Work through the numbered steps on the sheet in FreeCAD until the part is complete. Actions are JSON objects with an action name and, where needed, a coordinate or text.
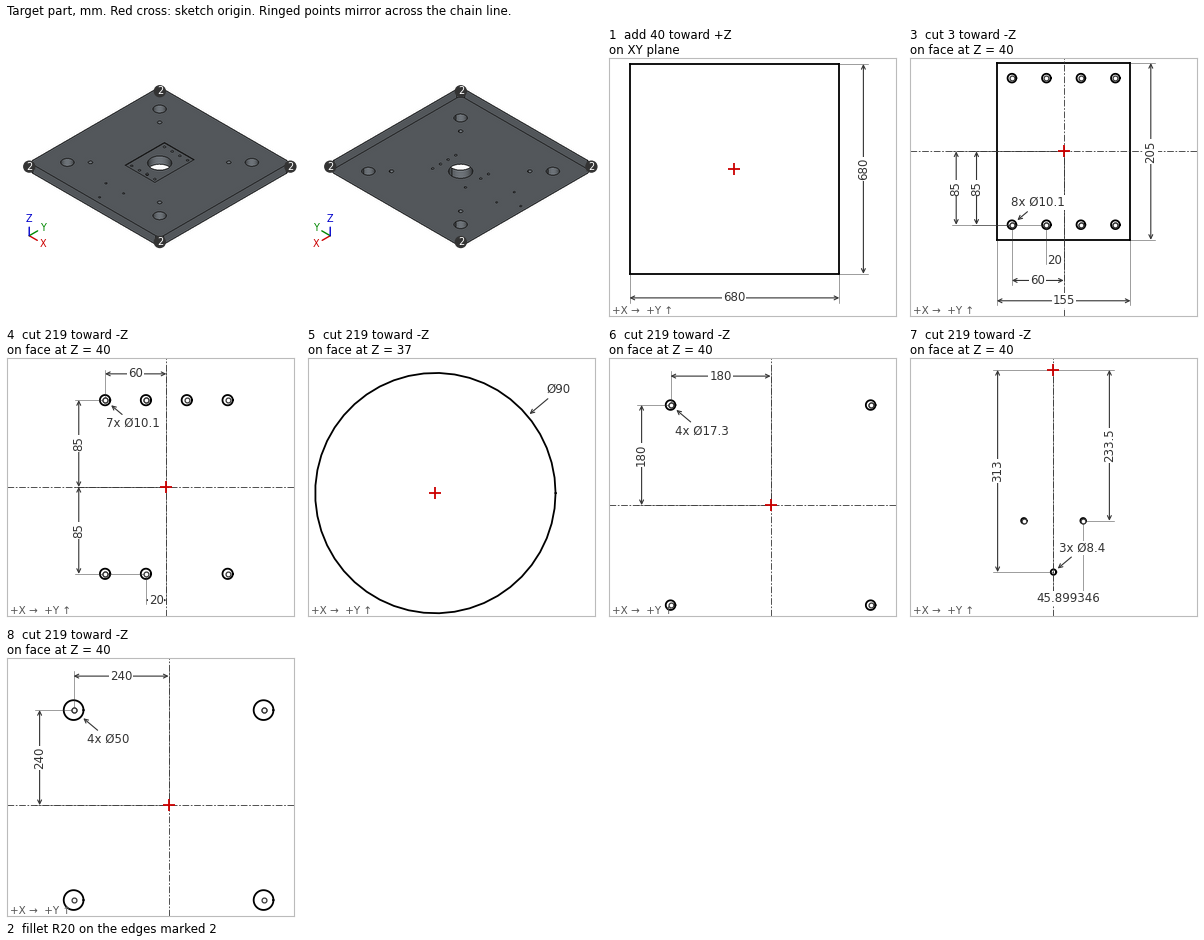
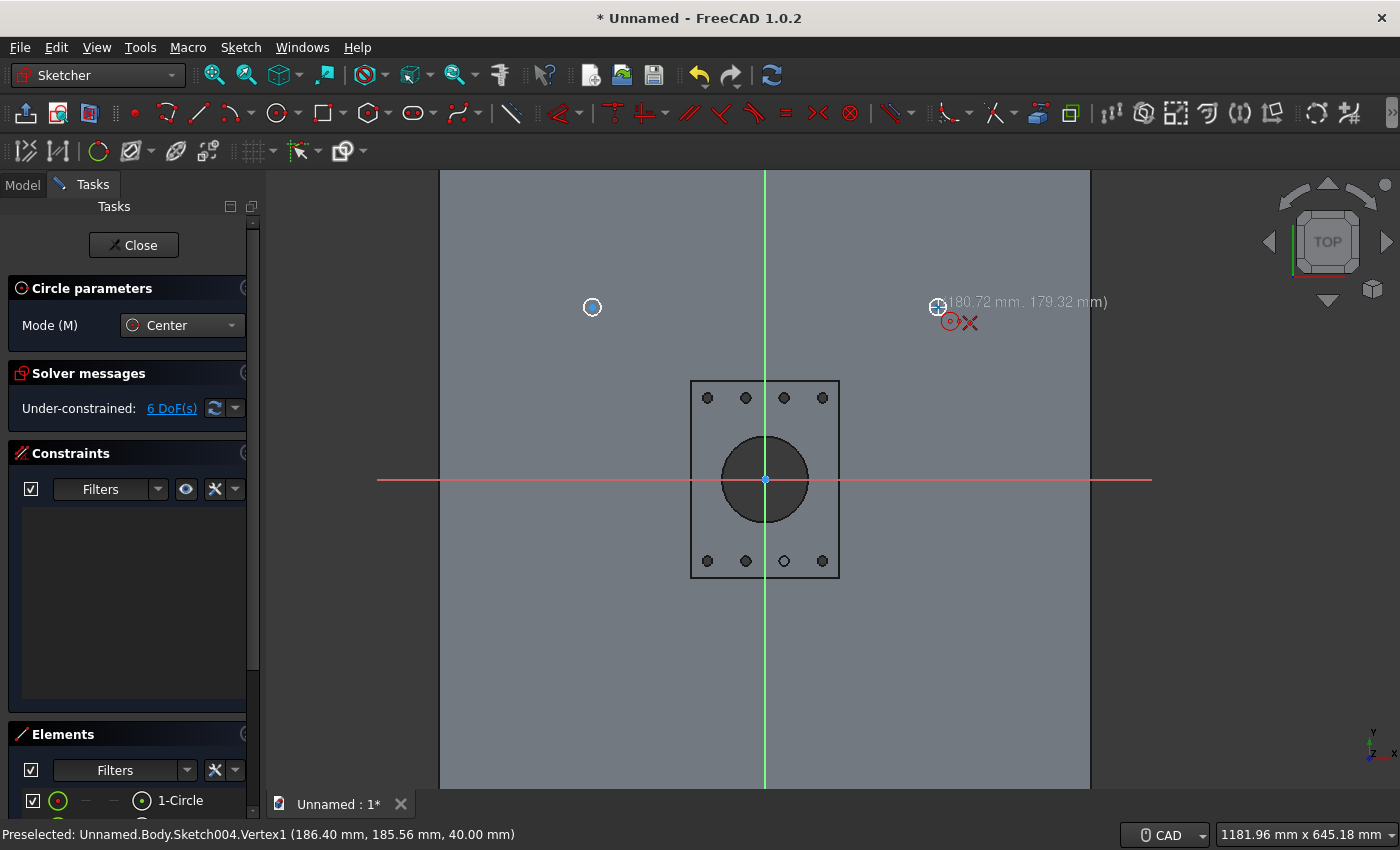
{"action": "scroll", "coordinate": [938, 652], "scroll_direction": "up", "scroll_amount": 6}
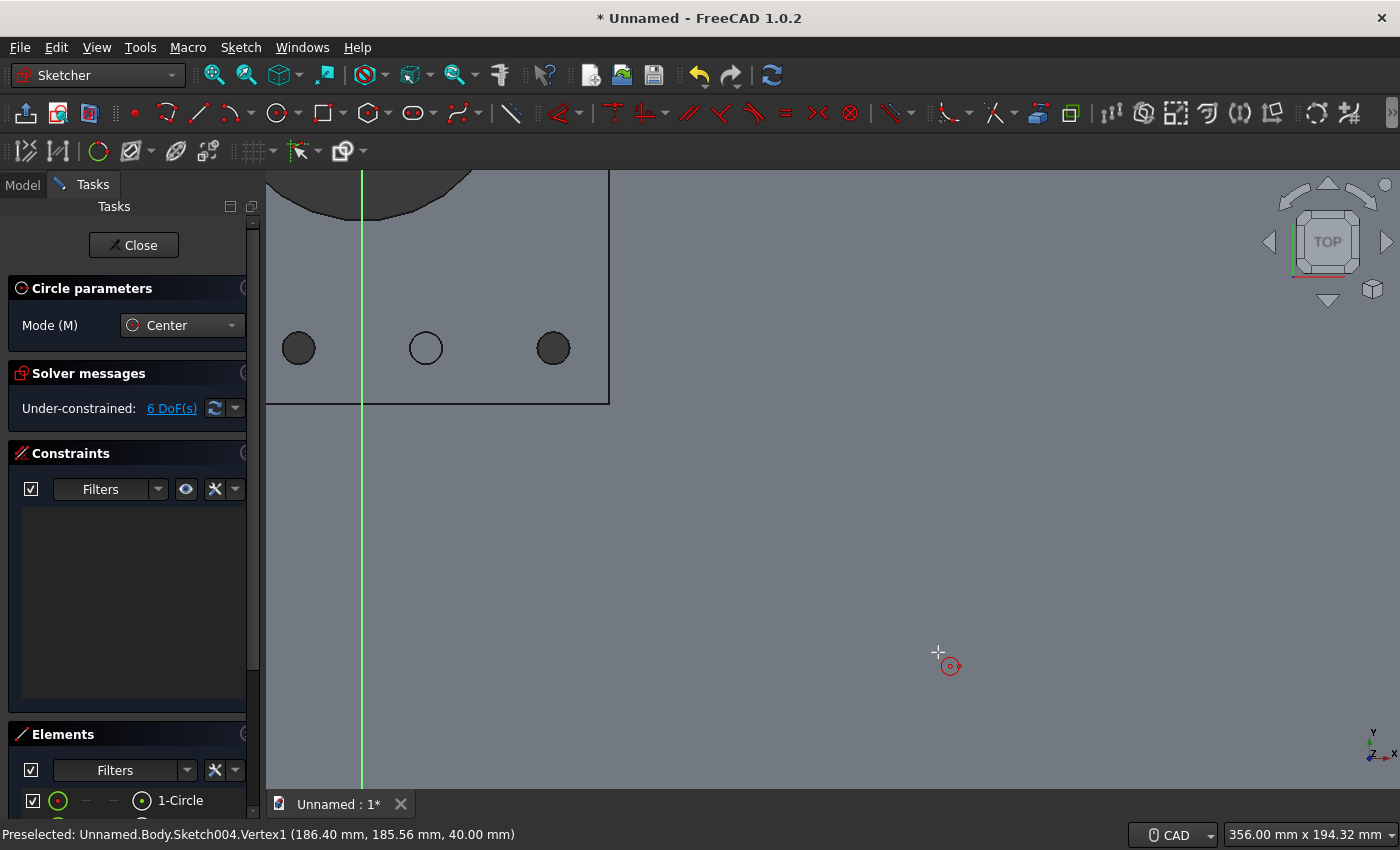
{"action": "left_click", "coordinate": [936, 651]}
{"action": "left_click", "coordinate": [955, 631]}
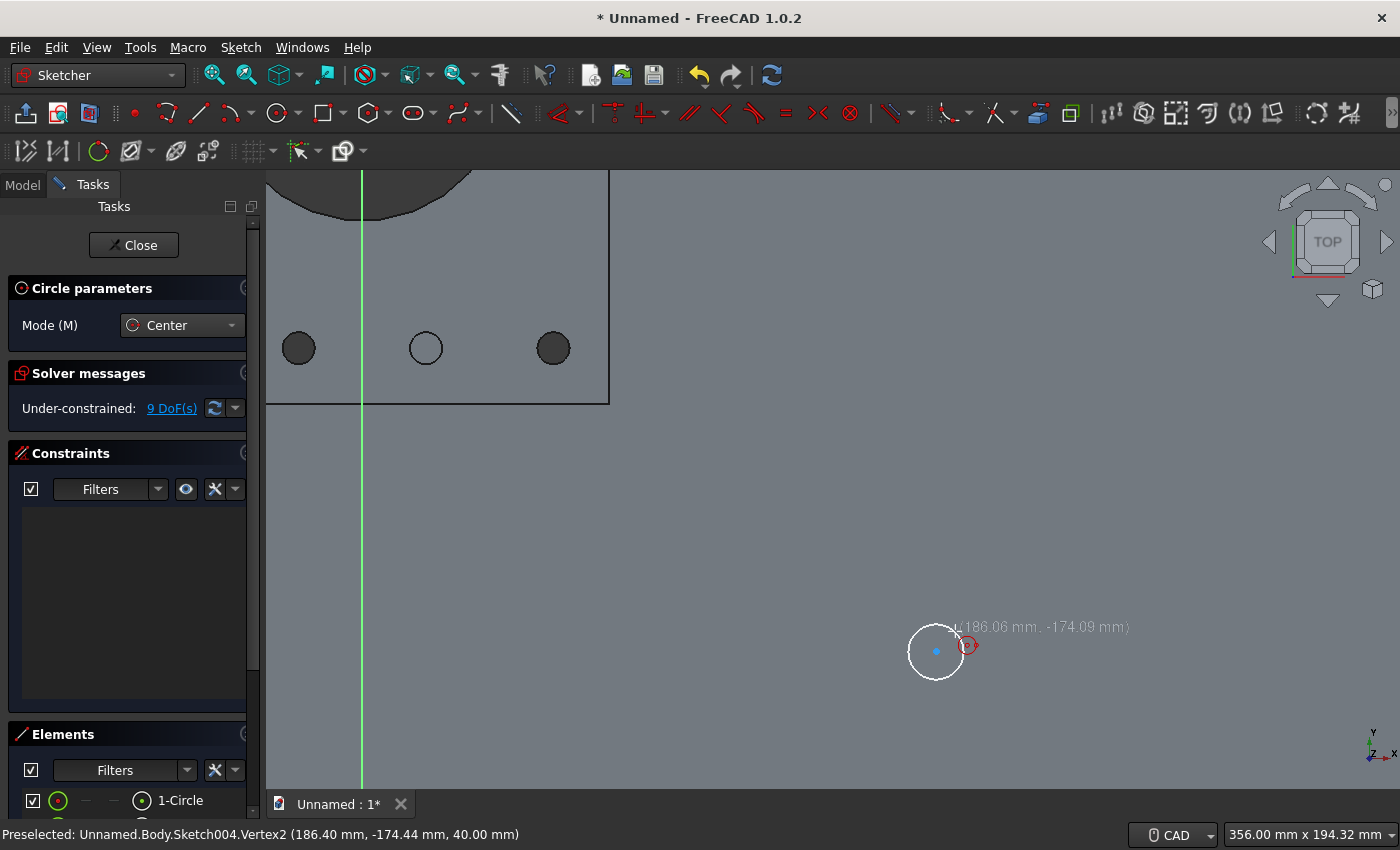
{"action": "scroll", "coordinate": [938, 653], "scroll_direction": "down", "scroll_amount": 6}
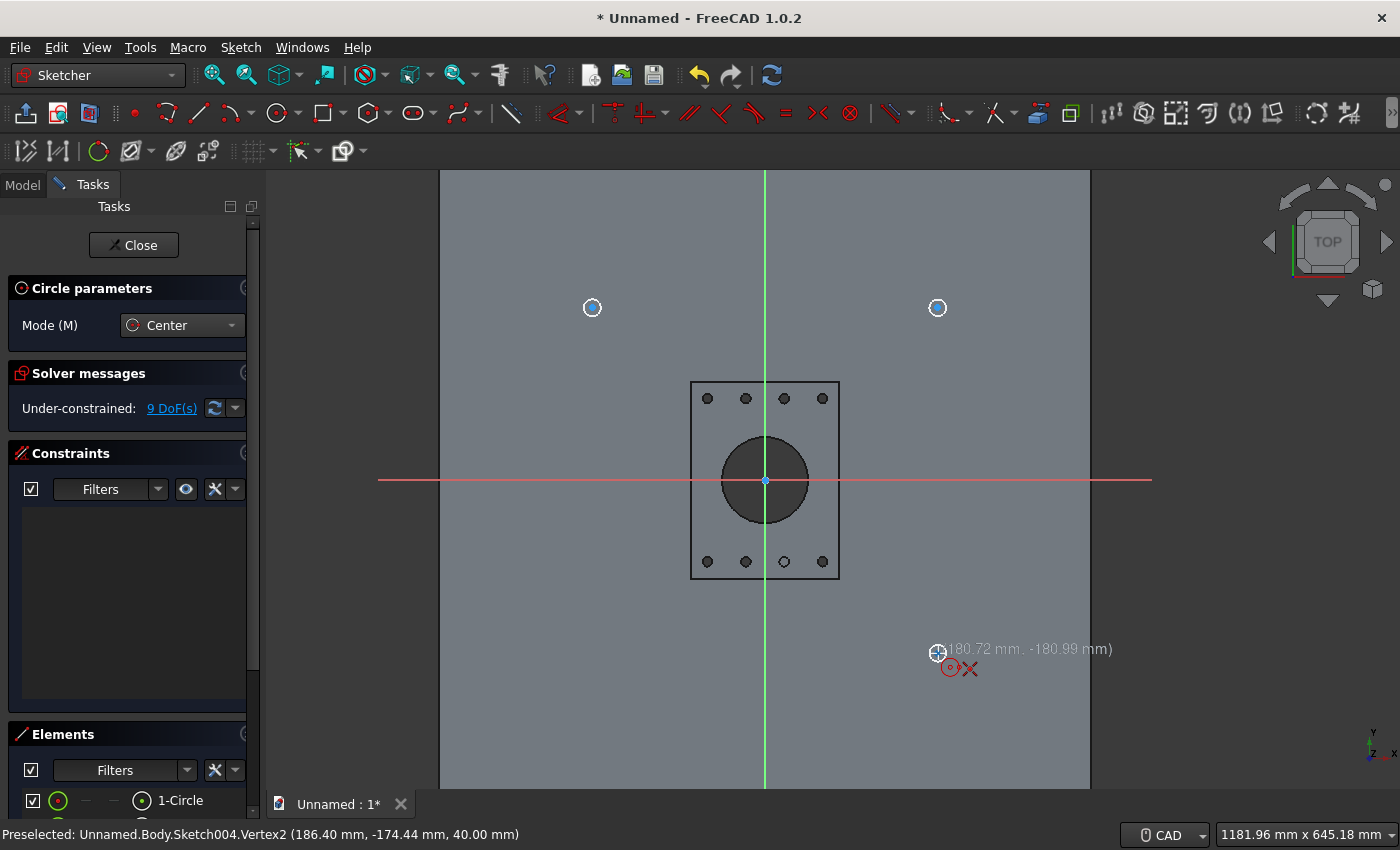
{"action": "scroll", "coordinate": [592, 653], "scroll_direction": "up", "scroll_amount": 6}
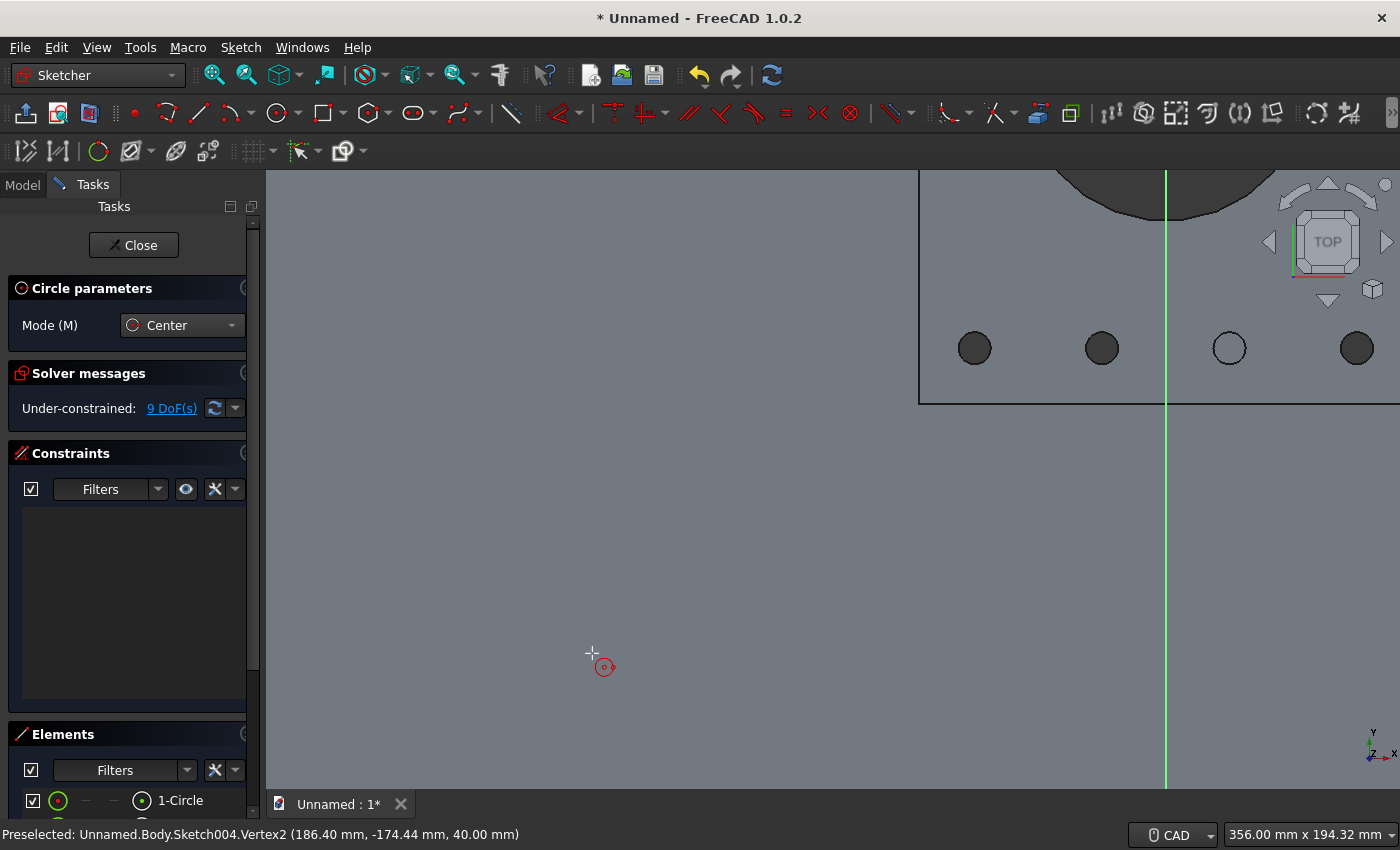
{"action": "left_click", "coordinate": [592, 651]}
{"action": "left_click", "coordinate": [612, 631]}
{"action": "key", "text": "Escape"}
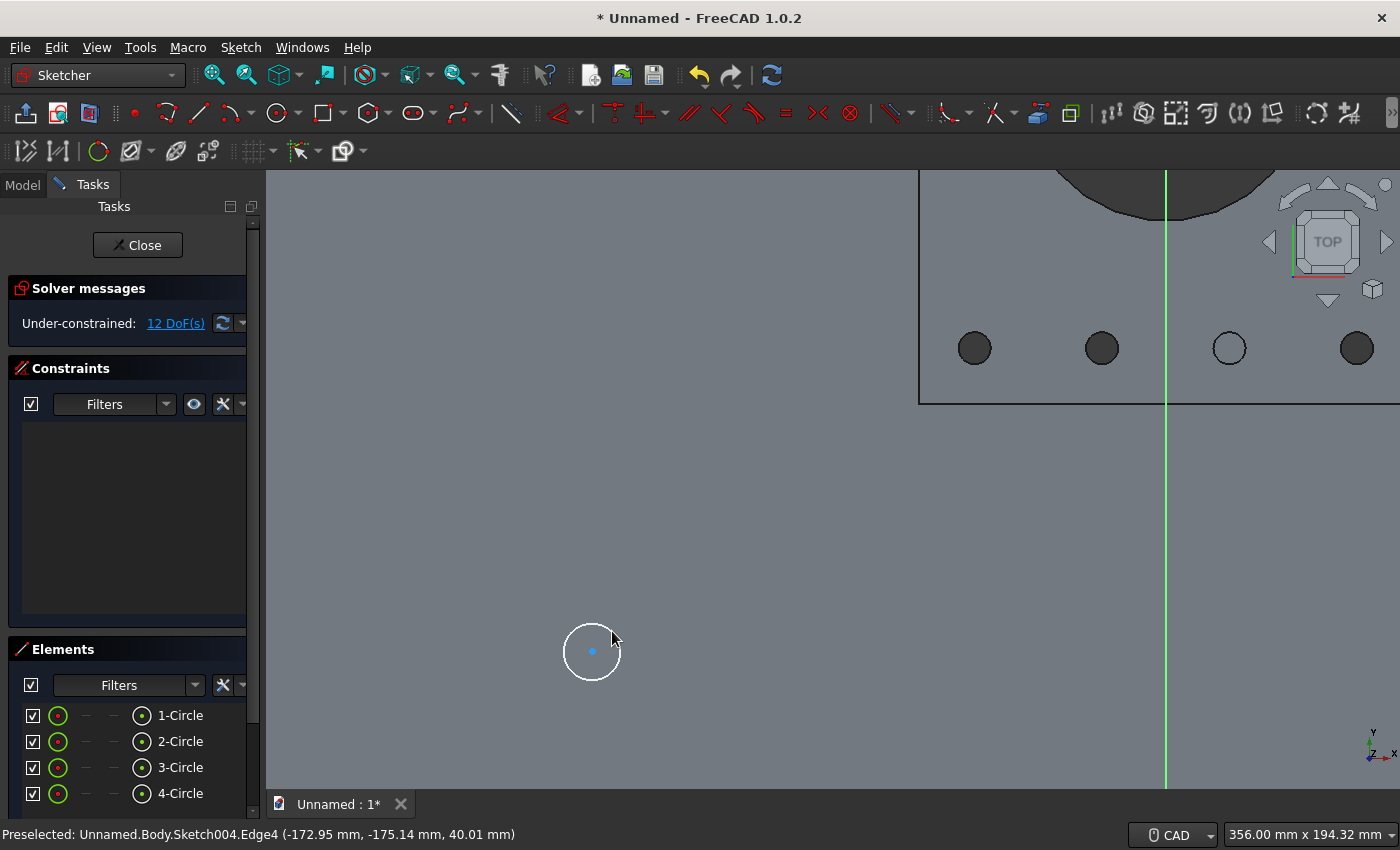
{"action": "scroll", "coordinate": [592, 653], "scroll_direction": "down", "scroll_amount": 6}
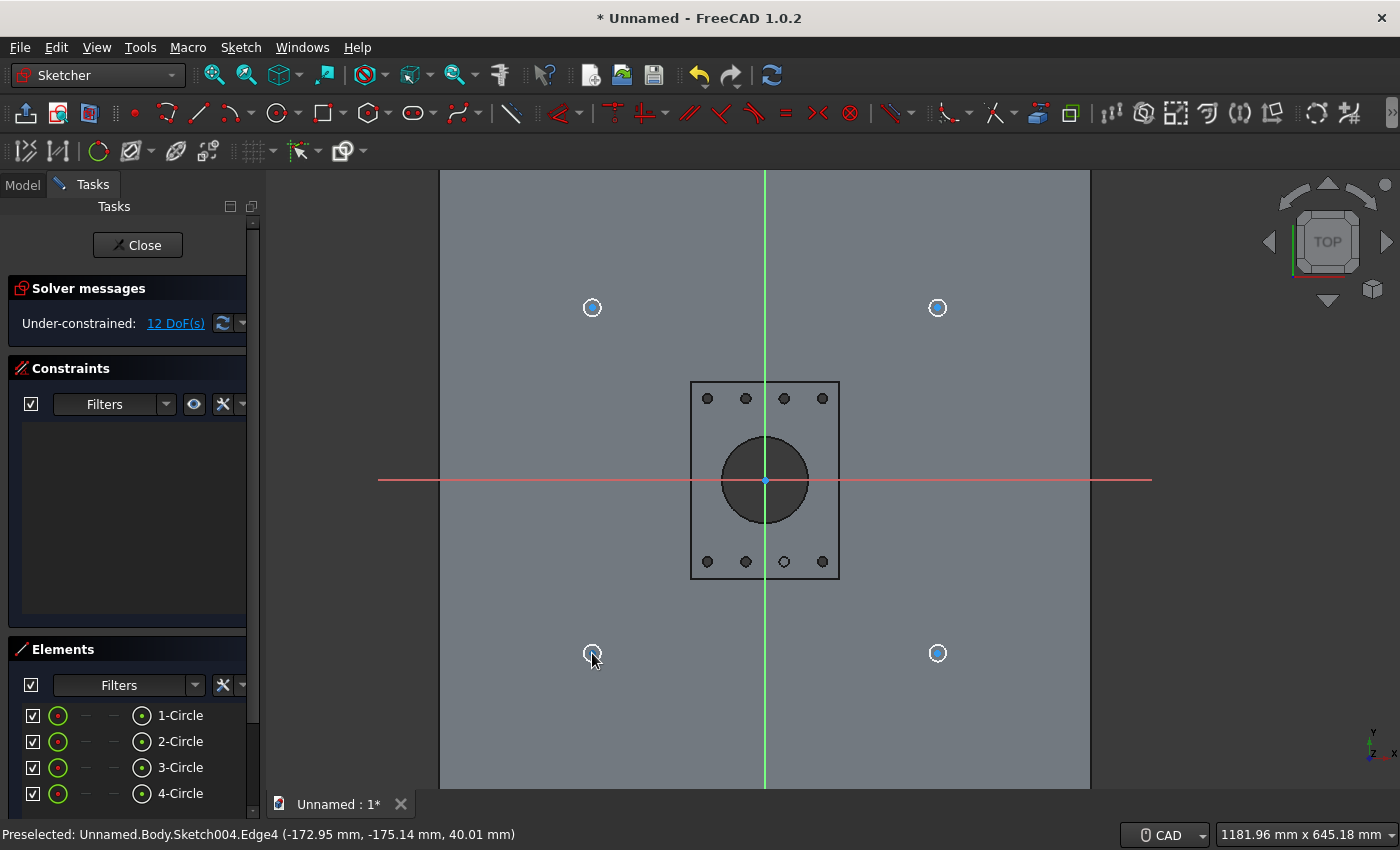
{"action": "scroll", "coordinate": [598, 302], "scroll_direction": "up", "scroll_amount": 3}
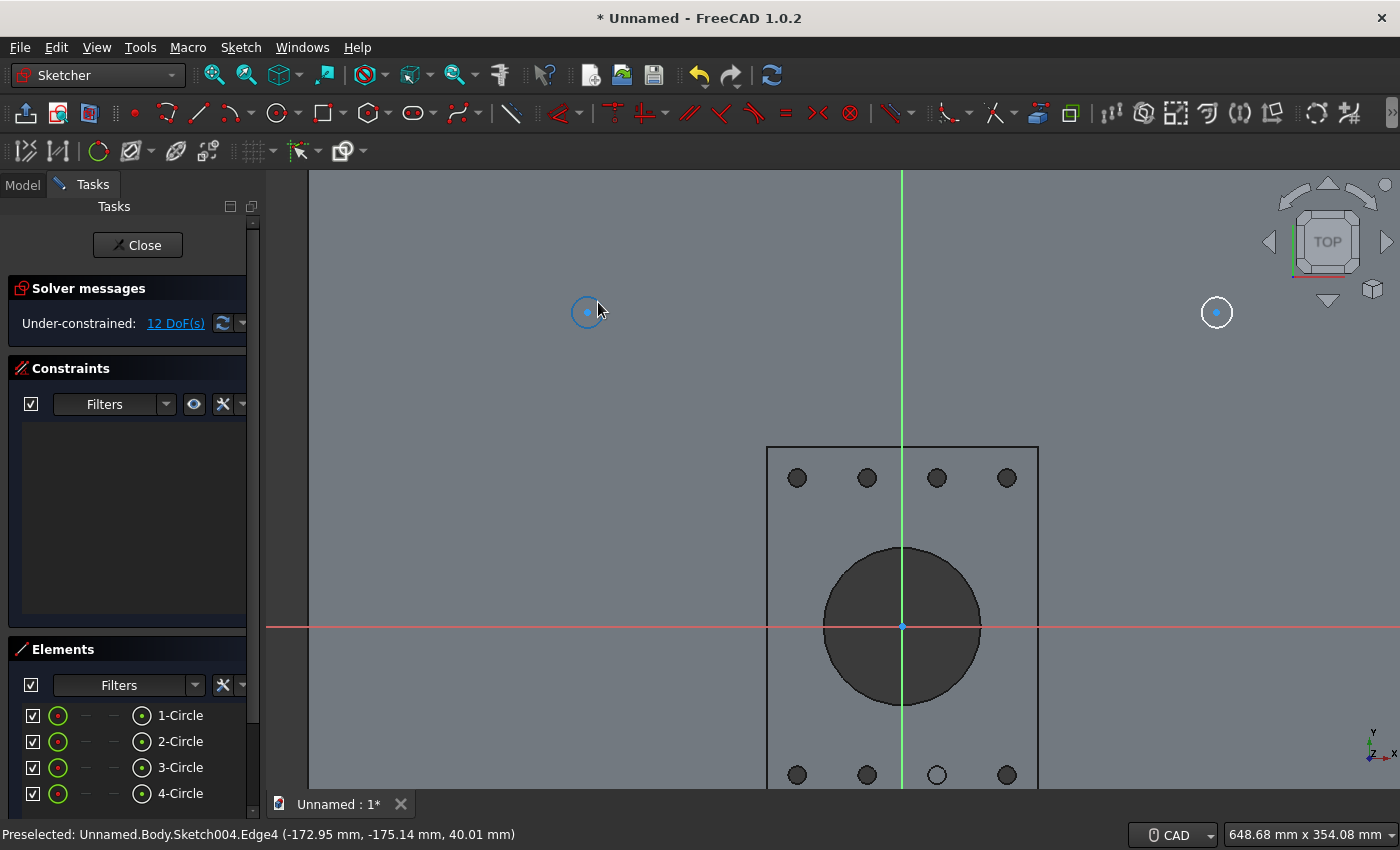
{"action": "left_click", "coordinate": [598, 301]}